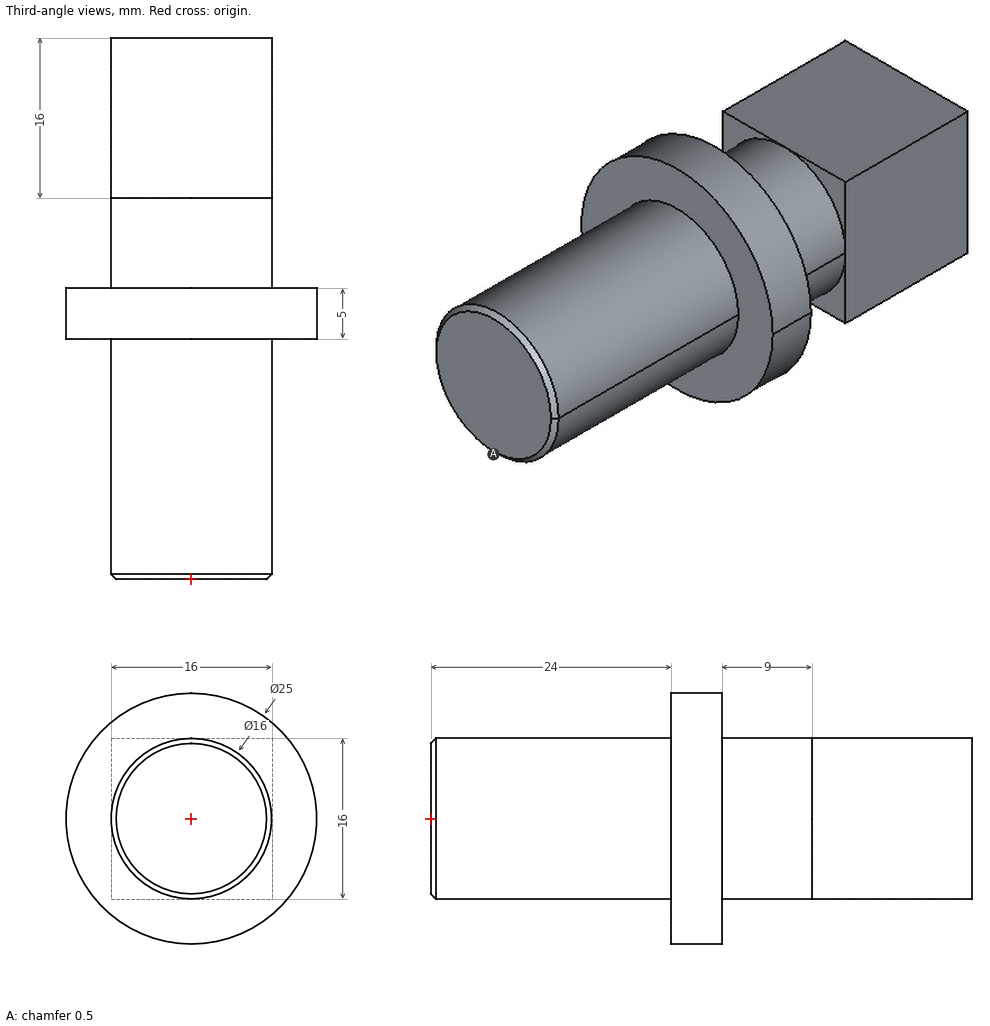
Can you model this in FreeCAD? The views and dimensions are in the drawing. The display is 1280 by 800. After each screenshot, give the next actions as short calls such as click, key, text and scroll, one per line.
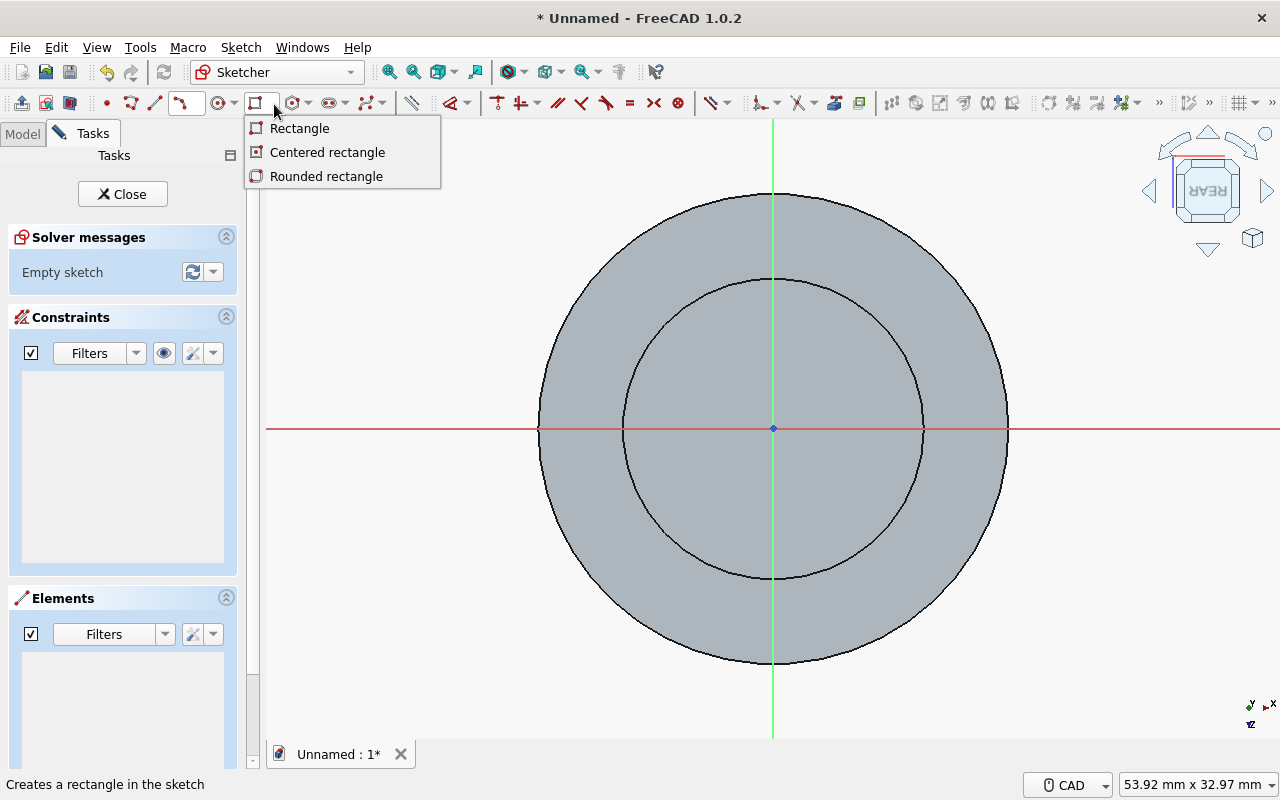
click(342, 152)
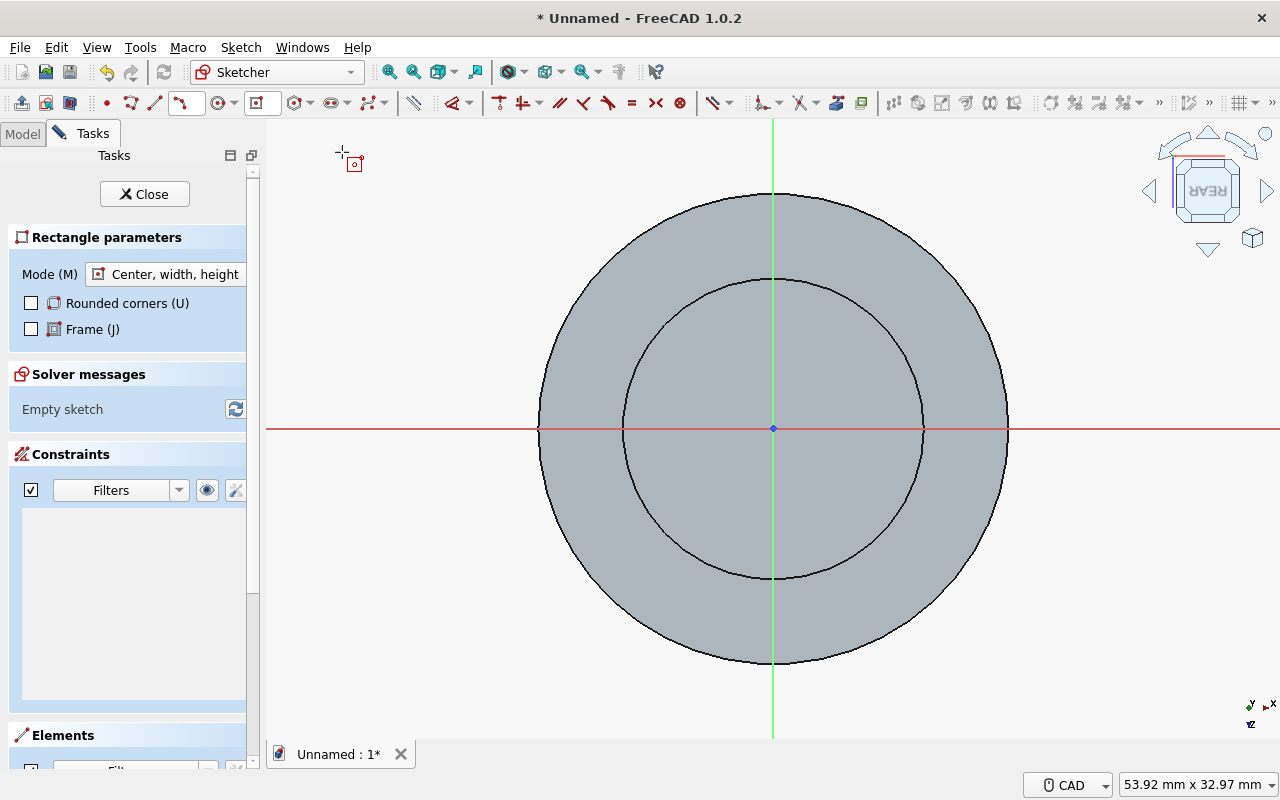
click(773, 429)
move(924, 279)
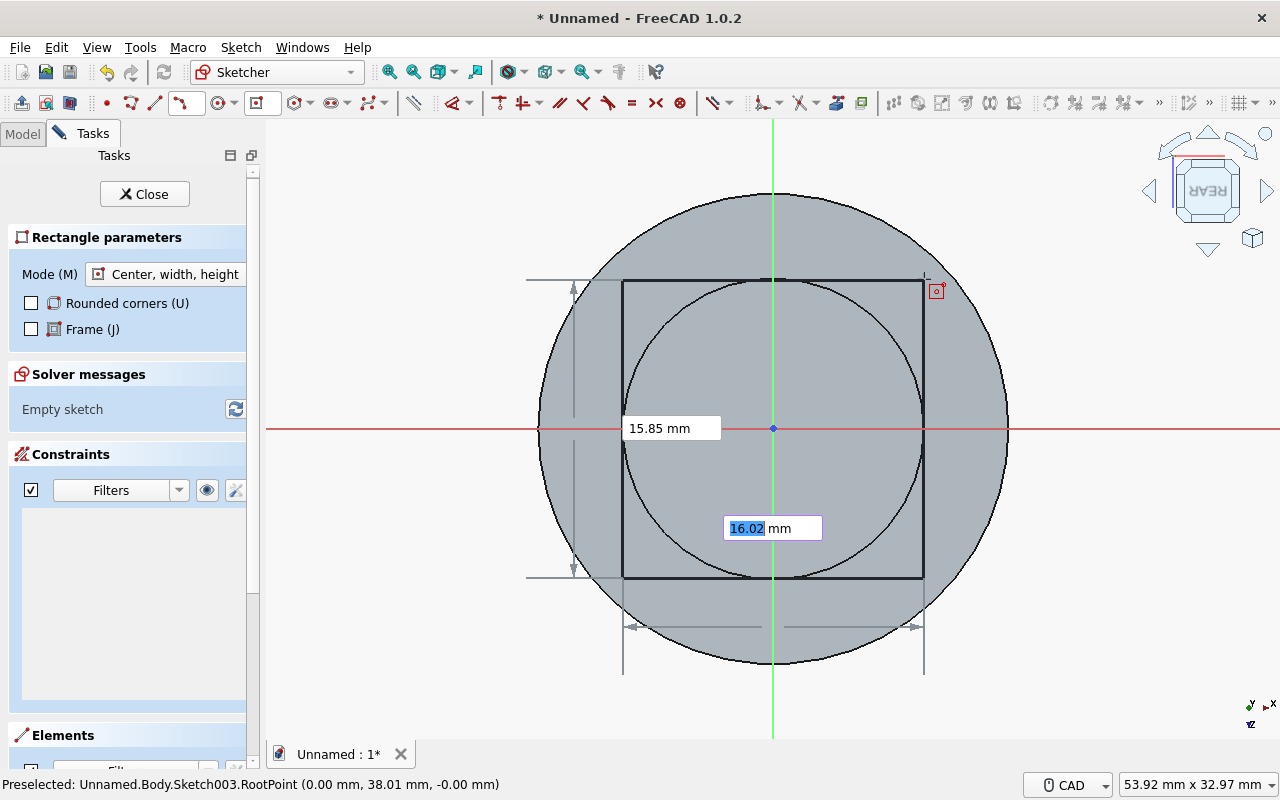
text(16)
key(Tab)
text(16)
key(Return)
key(Escape)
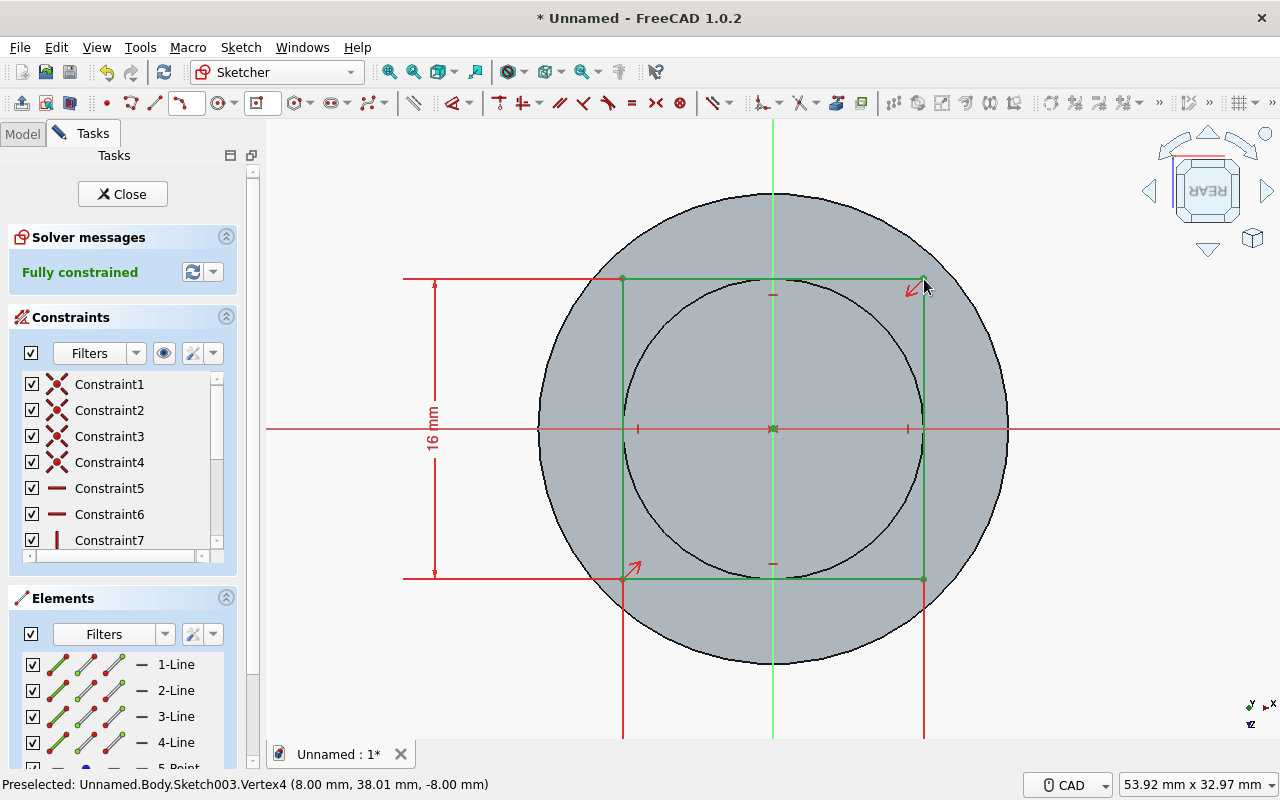
click(123, 194)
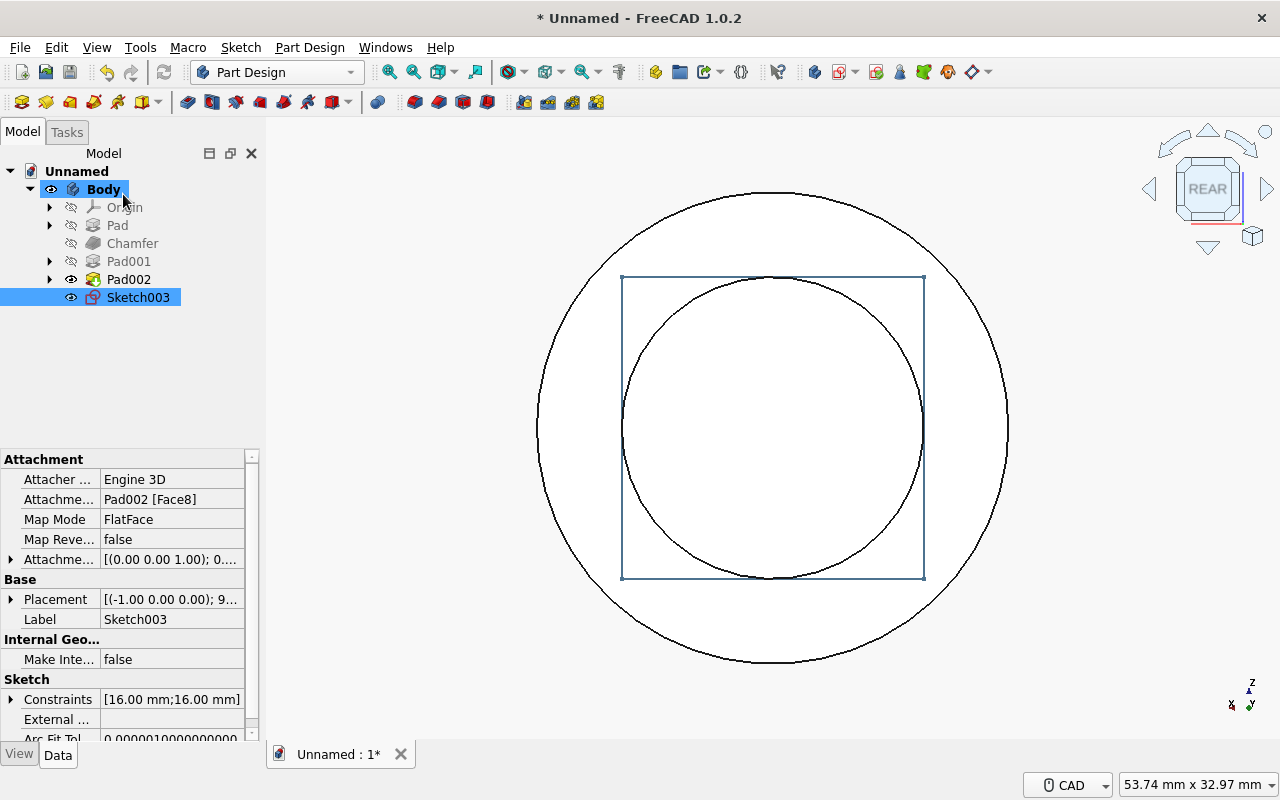
click(22, 102)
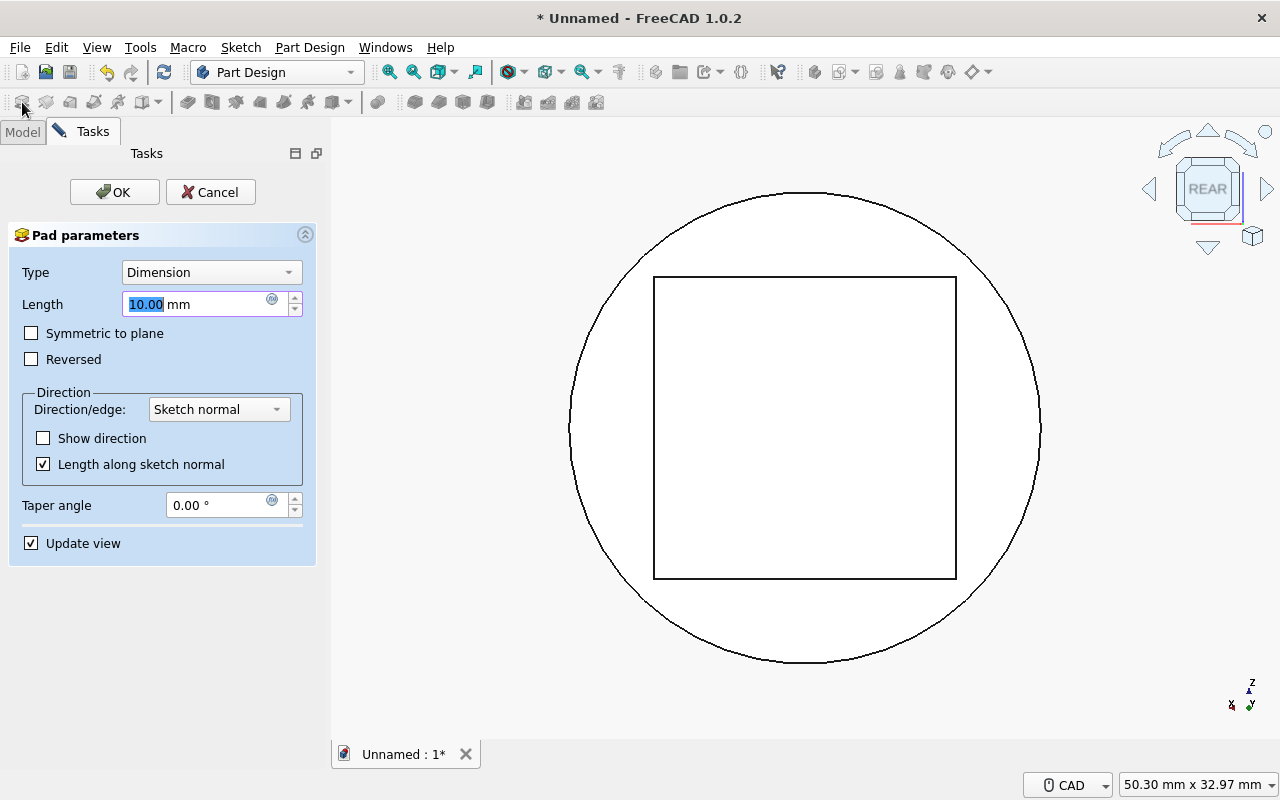
text(16)
key(Tab)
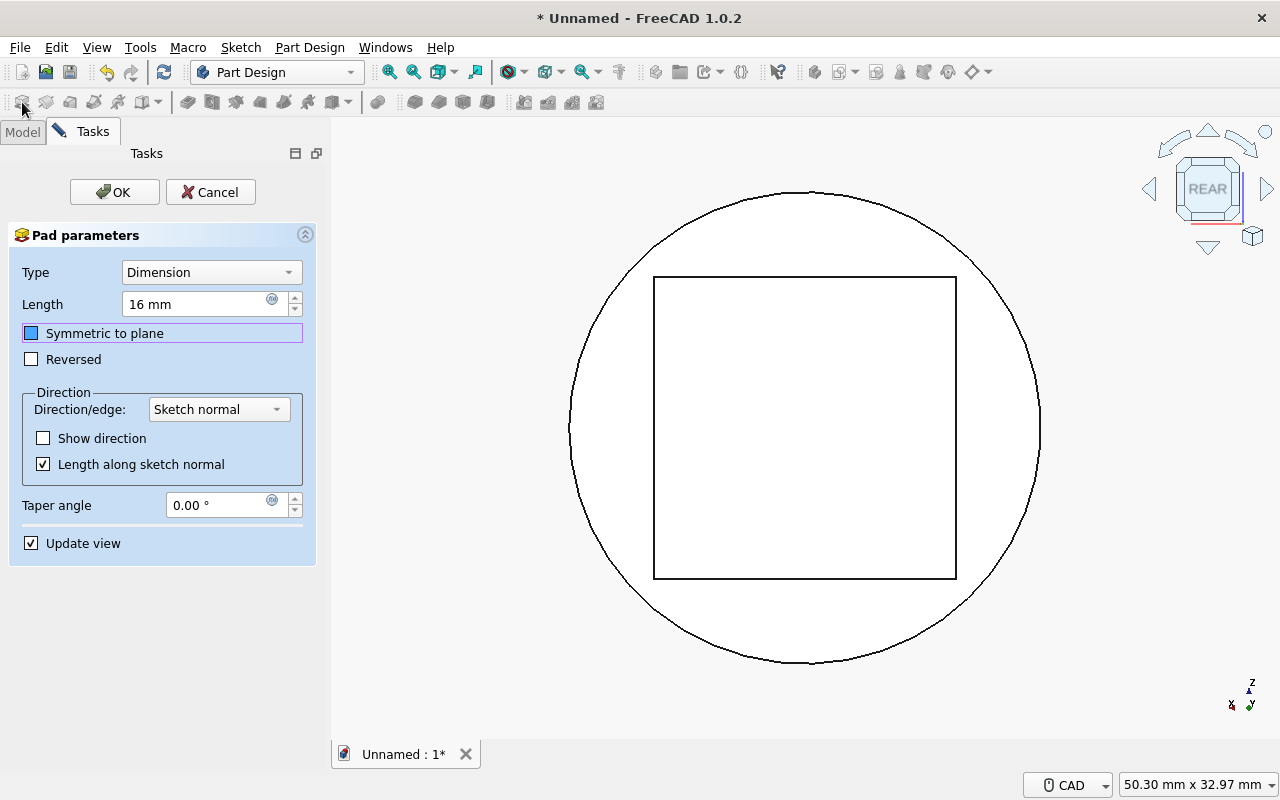
click(115, 192)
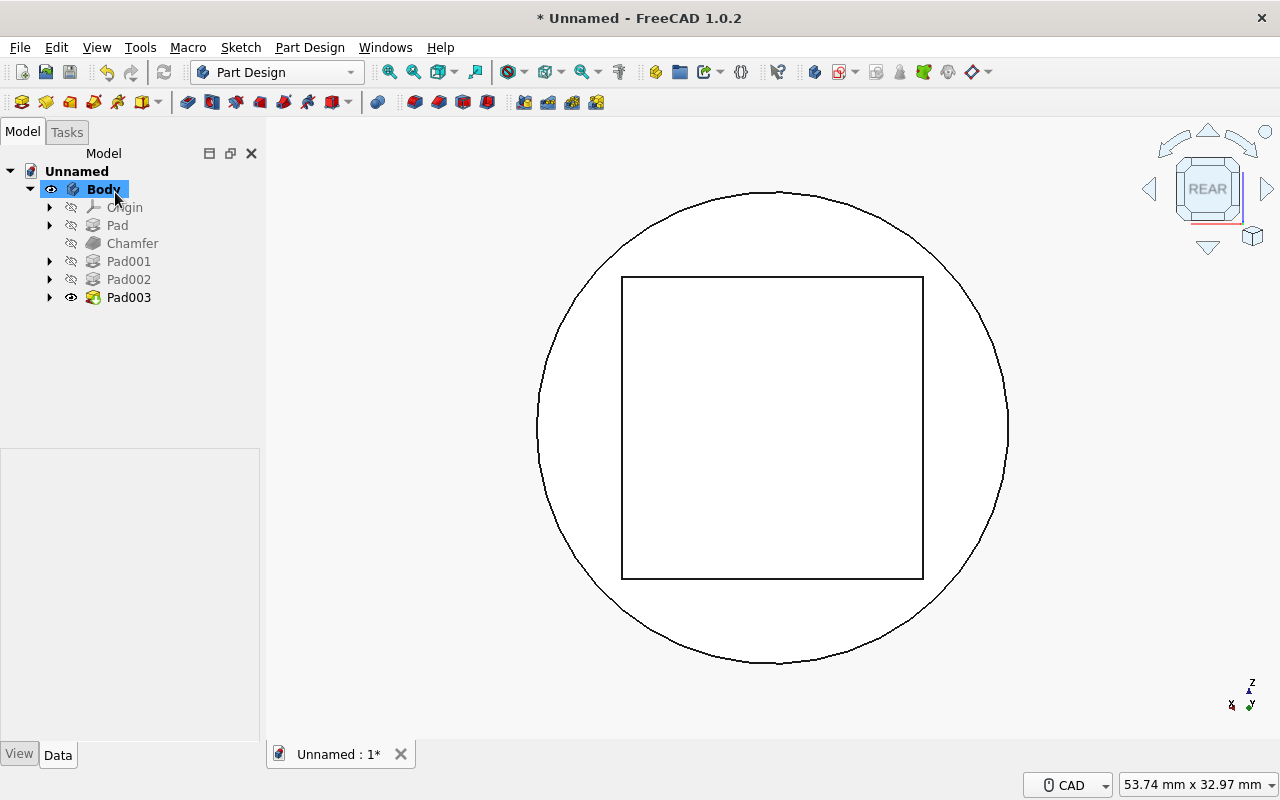
key(0)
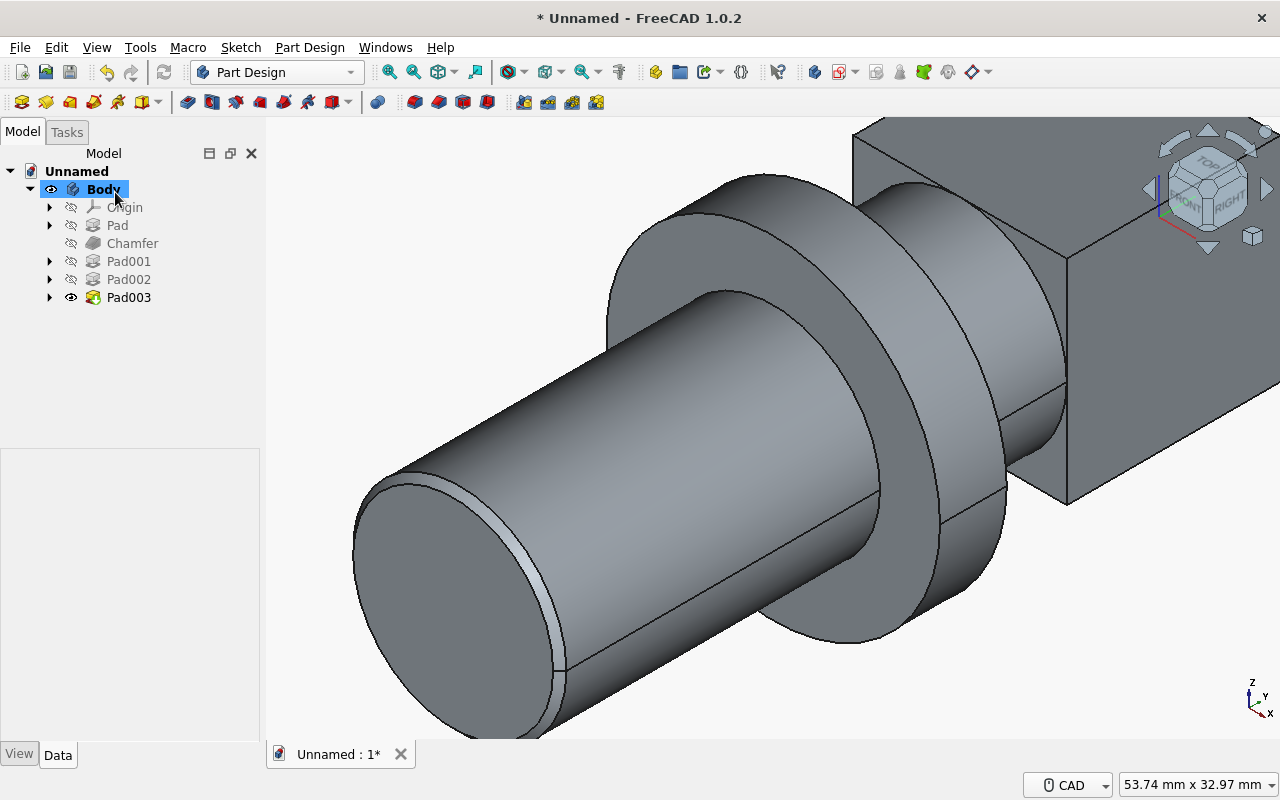
click(390, 72)